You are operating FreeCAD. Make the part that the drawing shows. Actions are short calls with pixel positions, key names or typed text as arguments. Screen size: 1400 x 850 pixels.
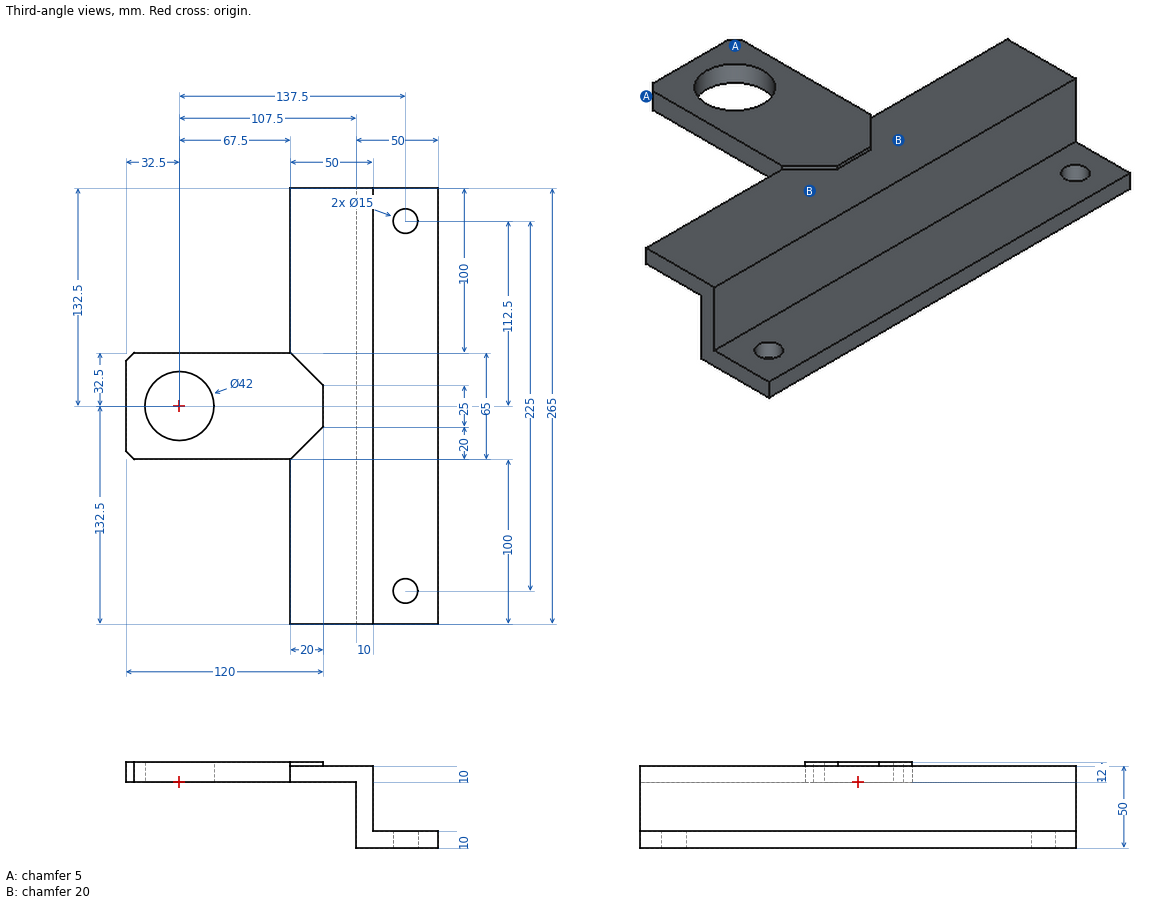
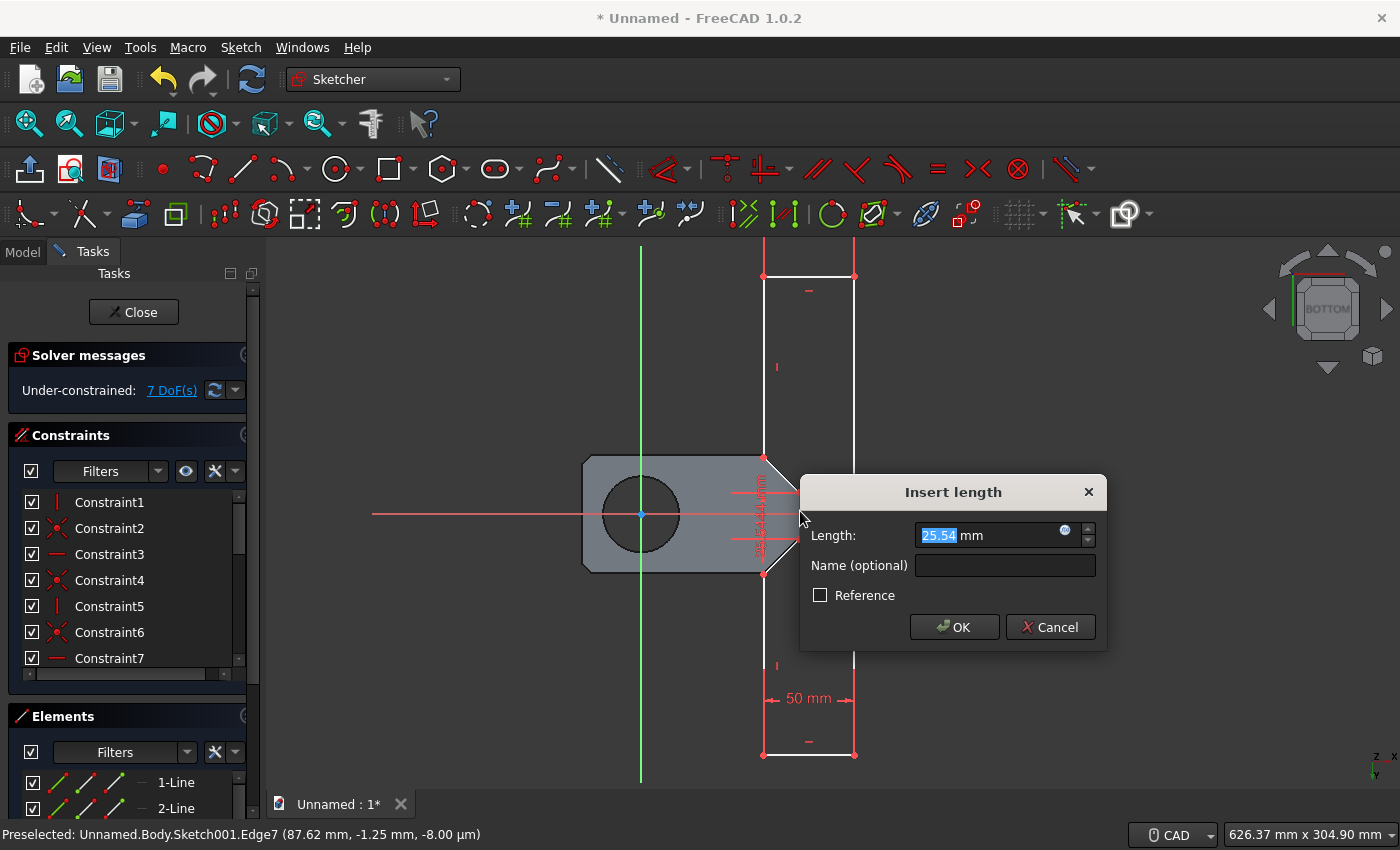
text(25)
key(Return)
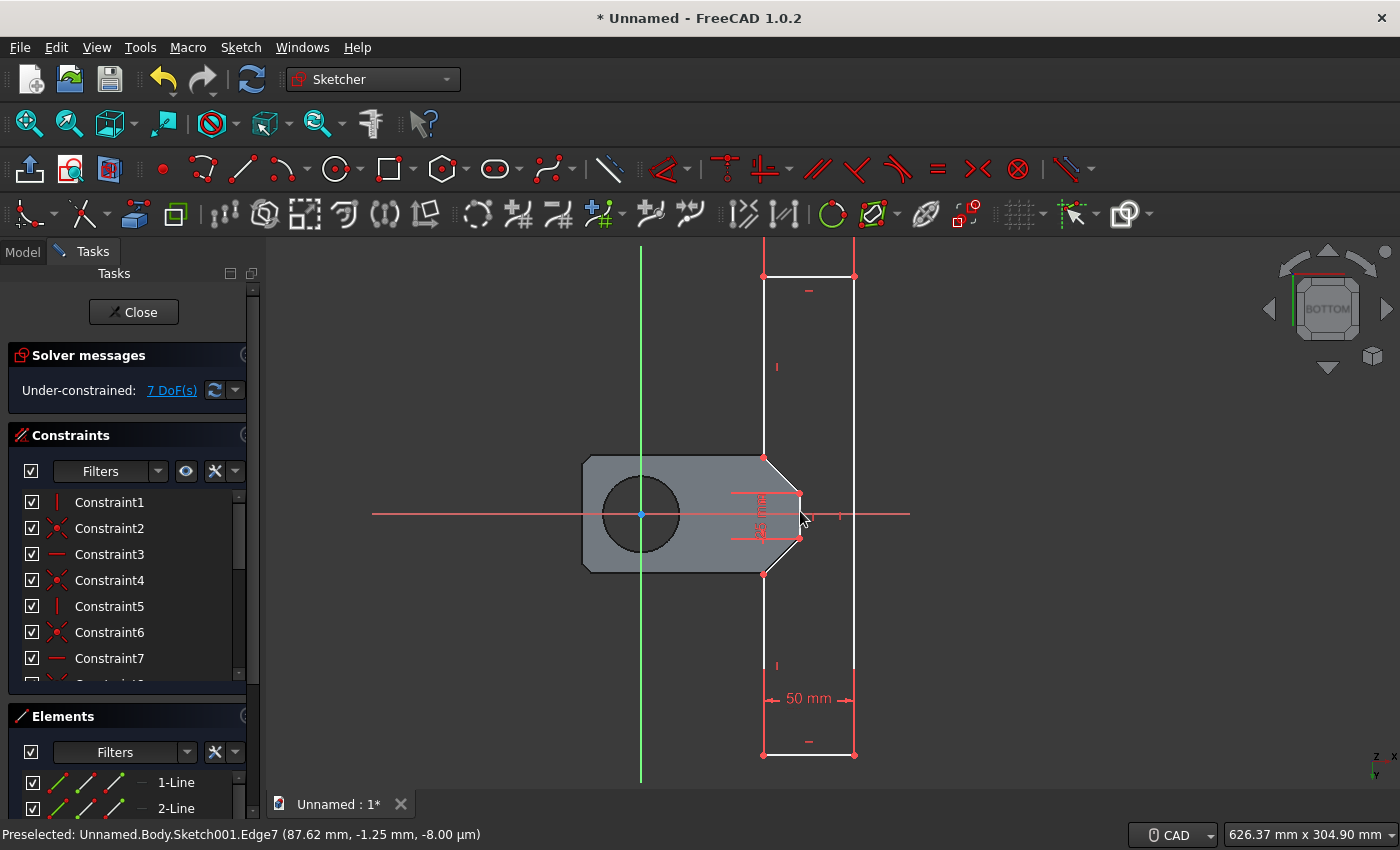
click(764, 629)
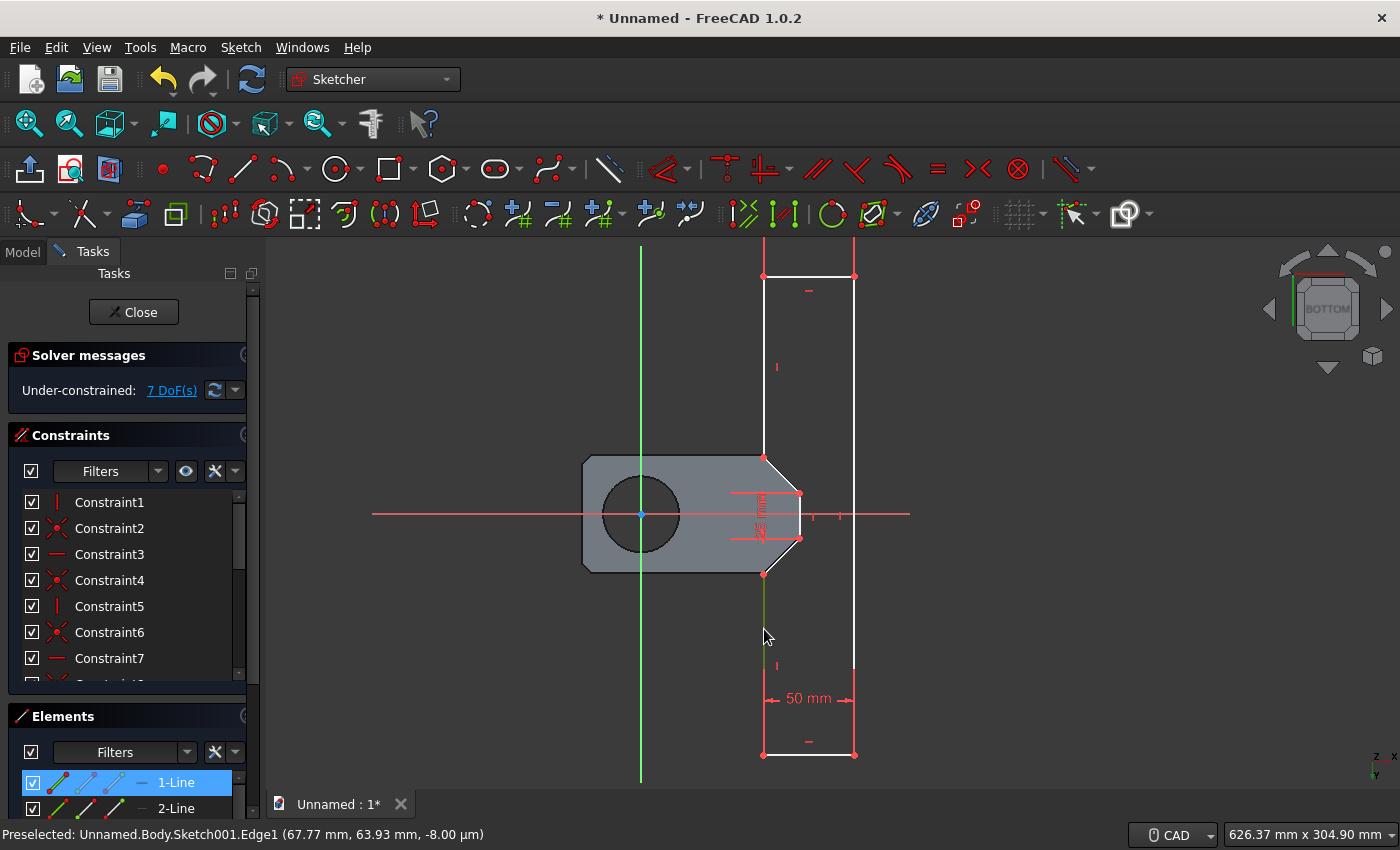
key(i)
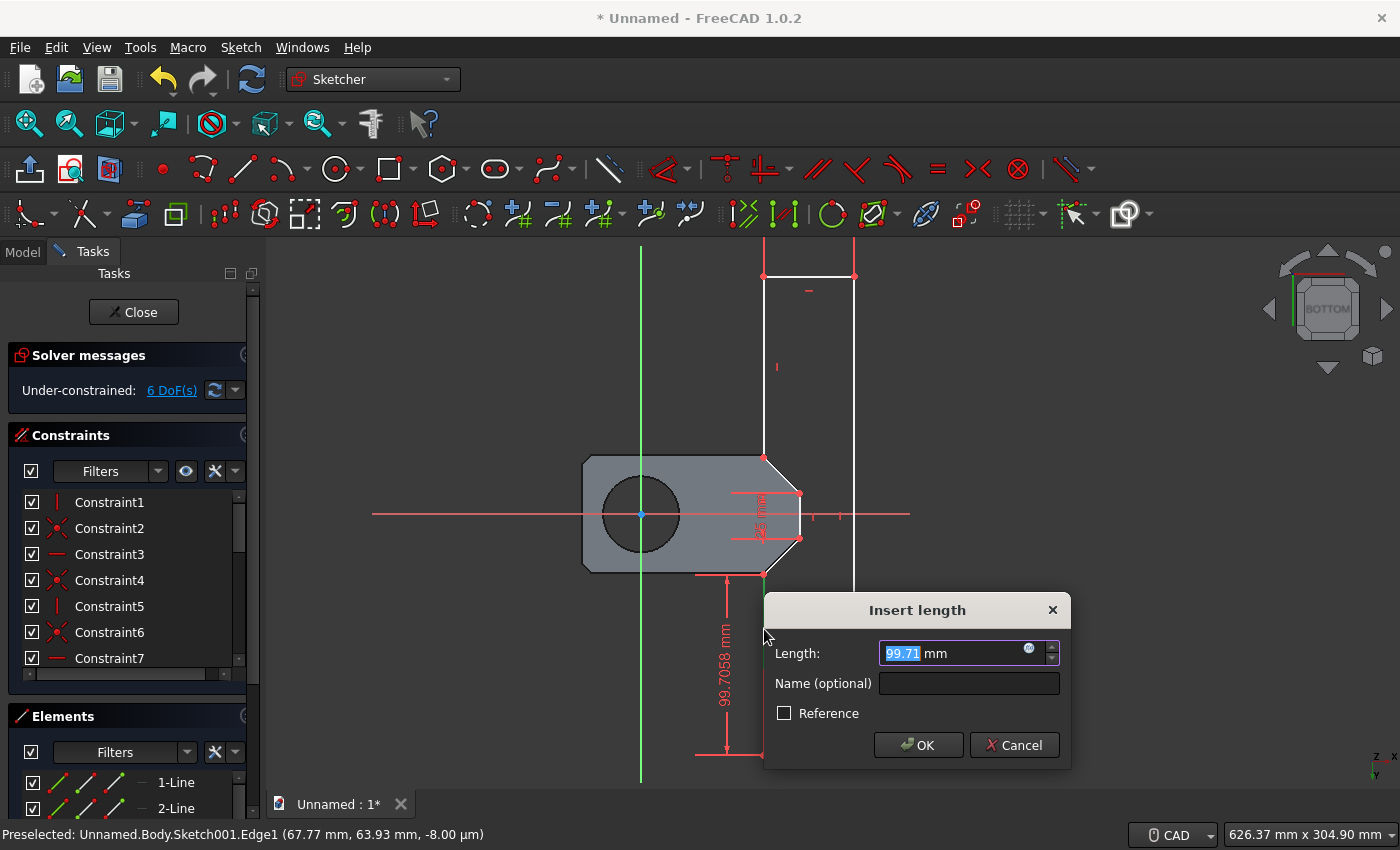
text(100)
key(Return)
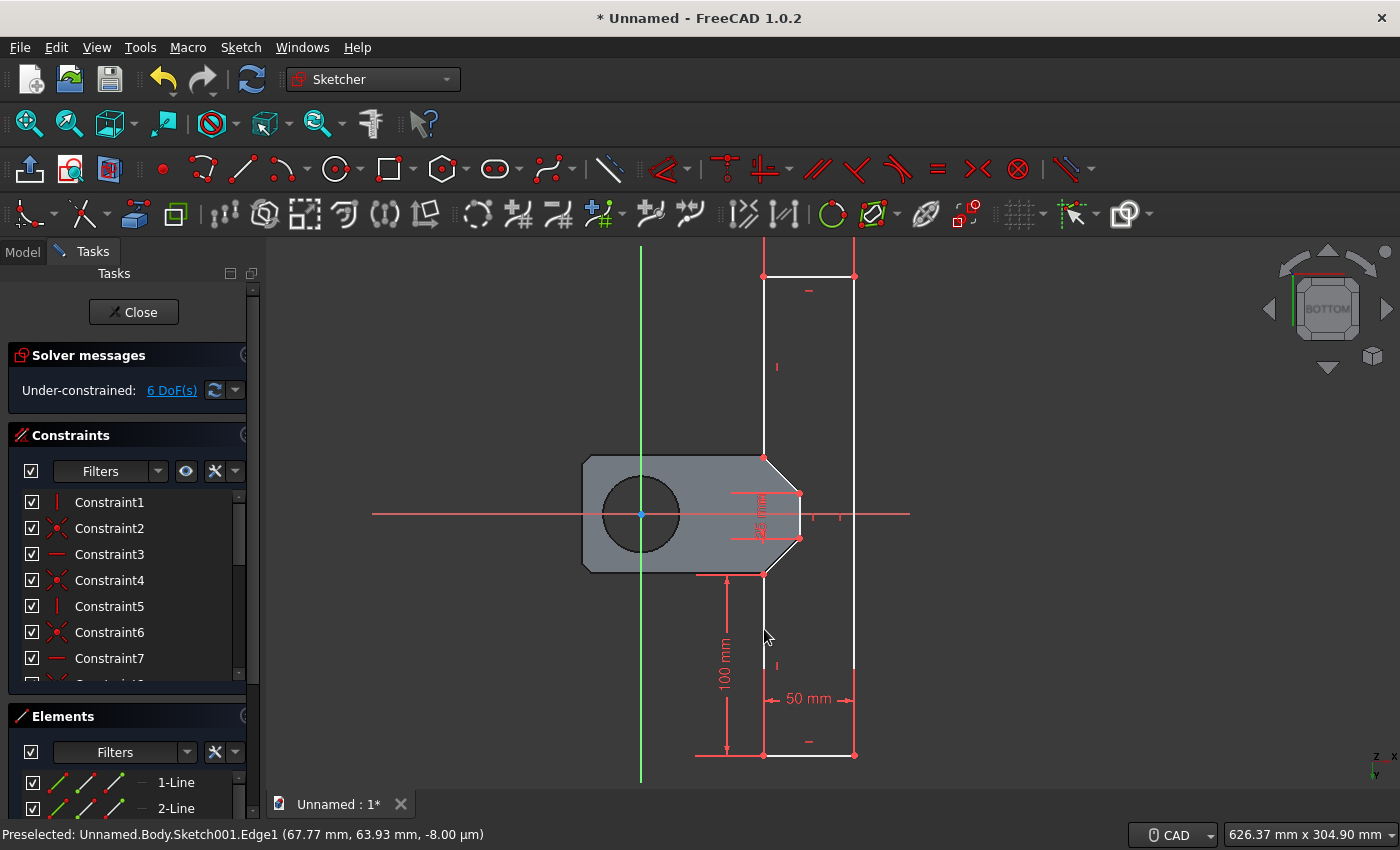
click(854, 612)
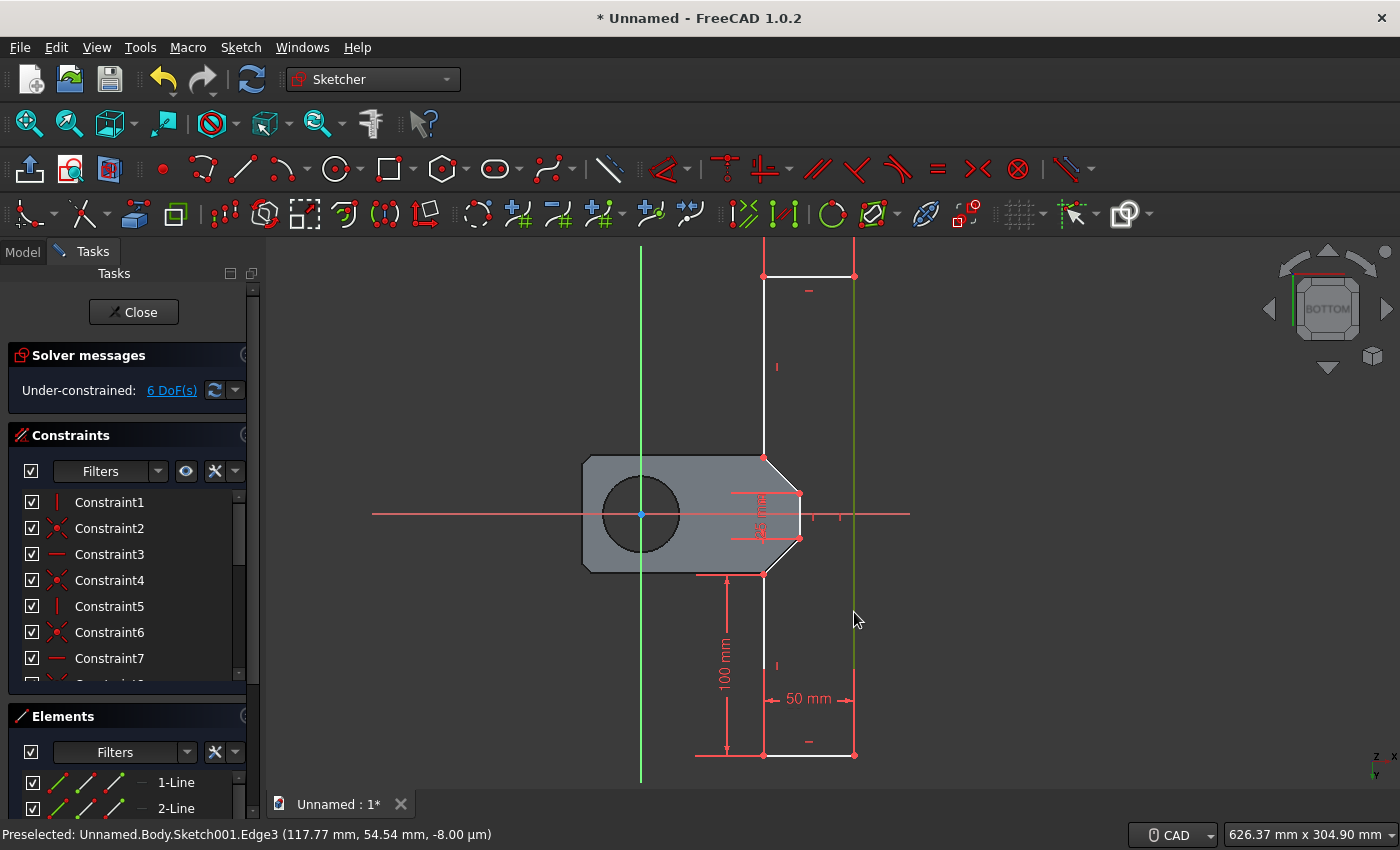
click(690, 170)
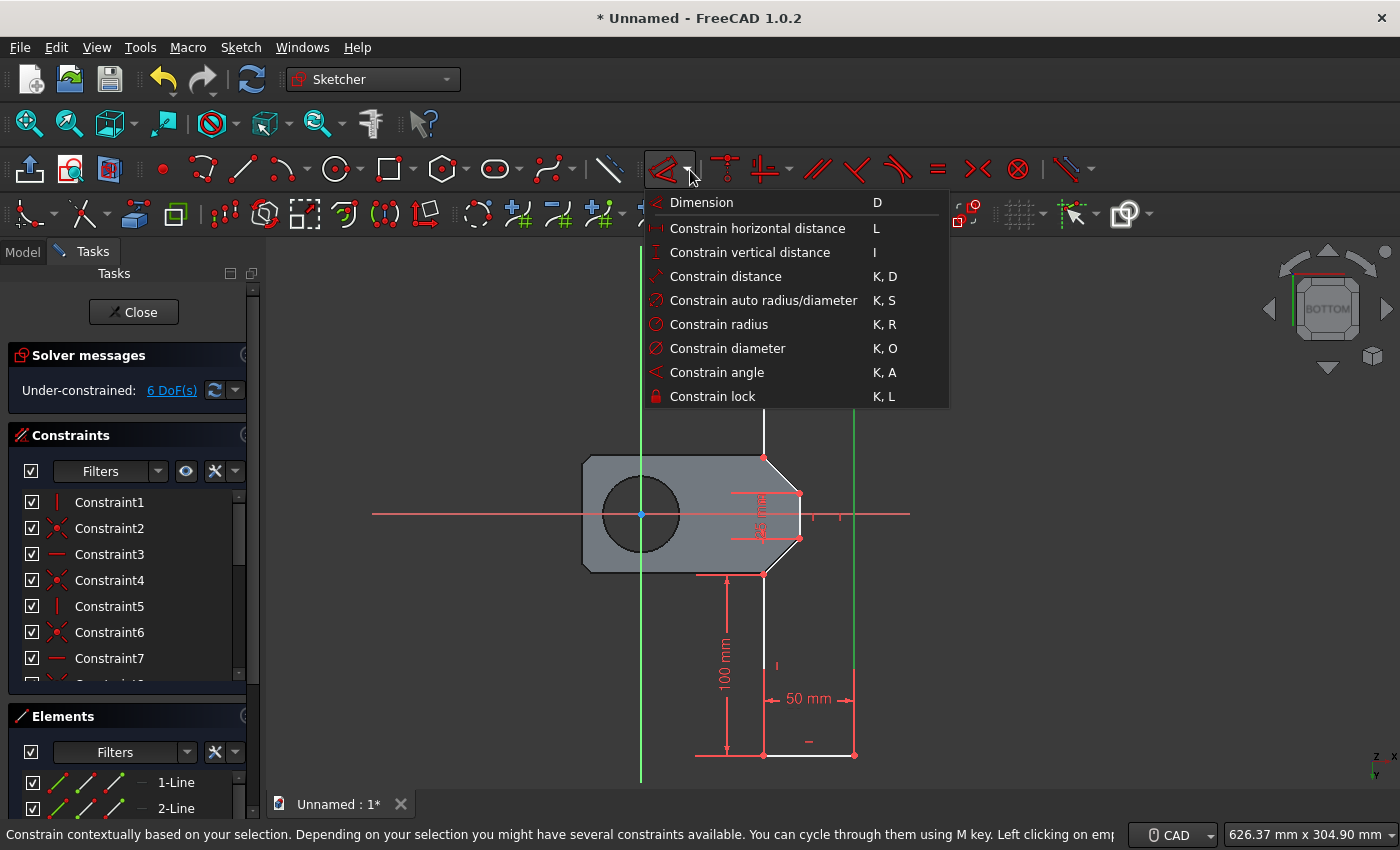
click(797, 252)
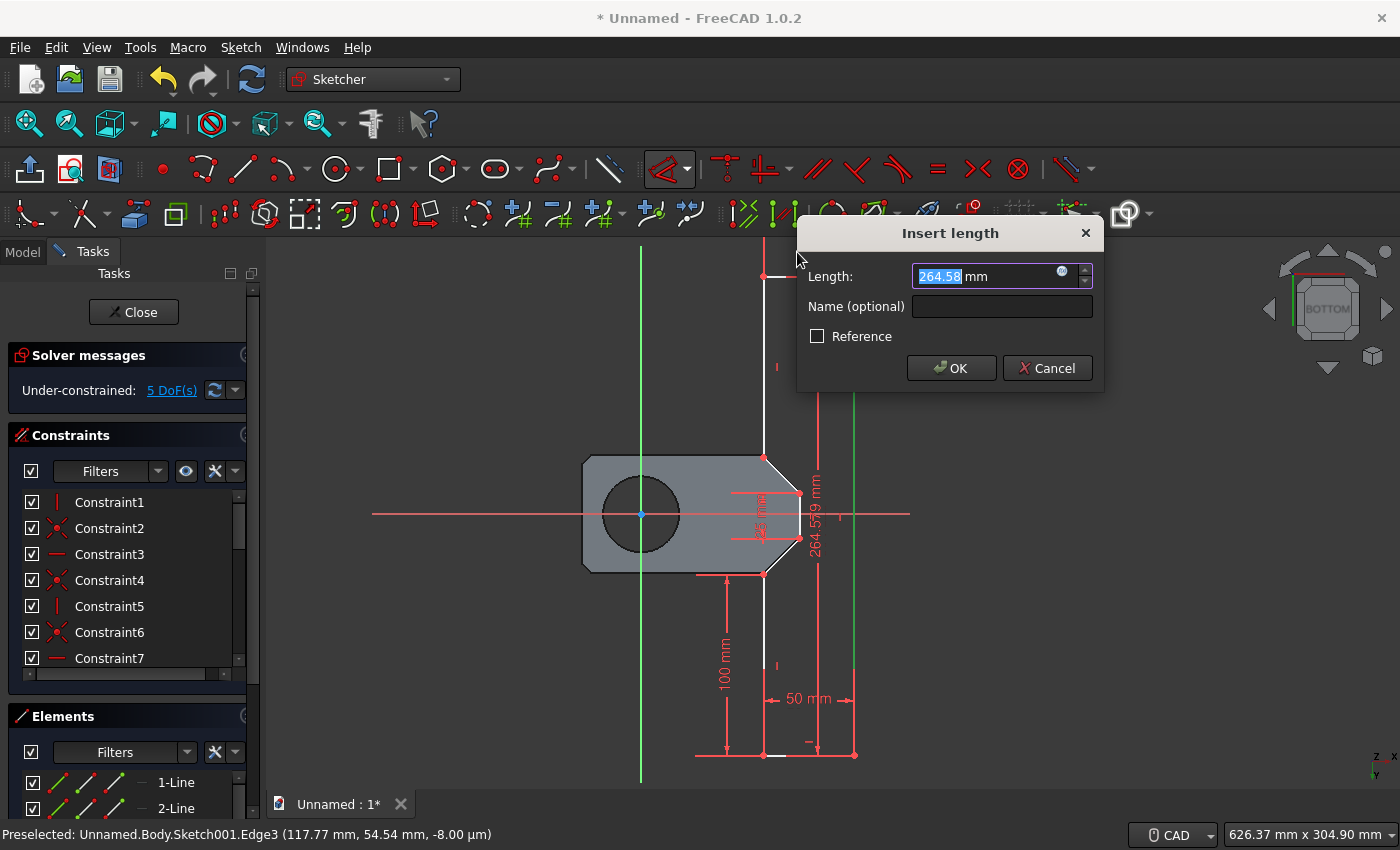
text(265)
key(Return)